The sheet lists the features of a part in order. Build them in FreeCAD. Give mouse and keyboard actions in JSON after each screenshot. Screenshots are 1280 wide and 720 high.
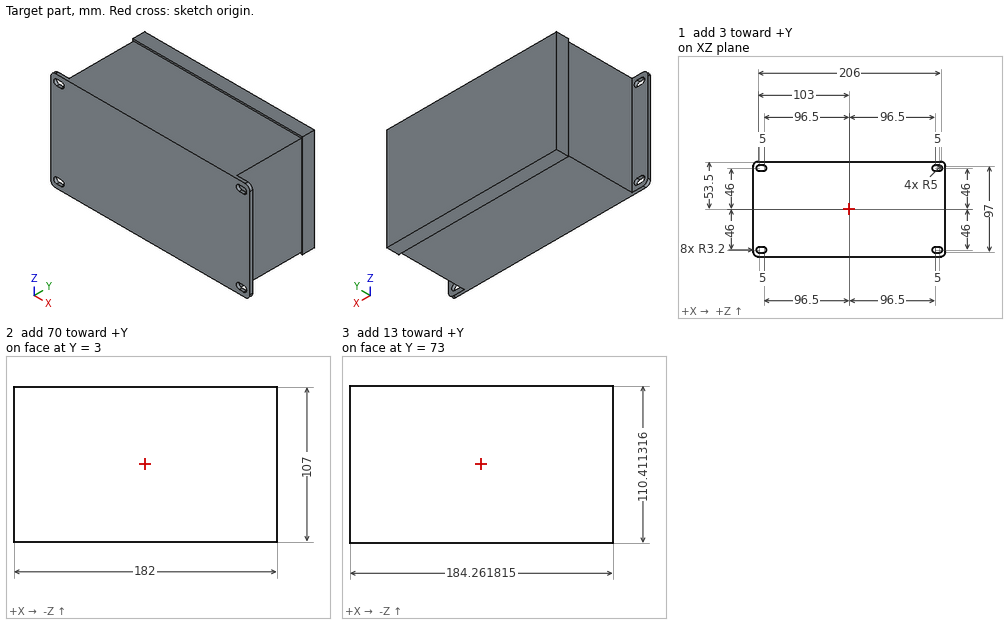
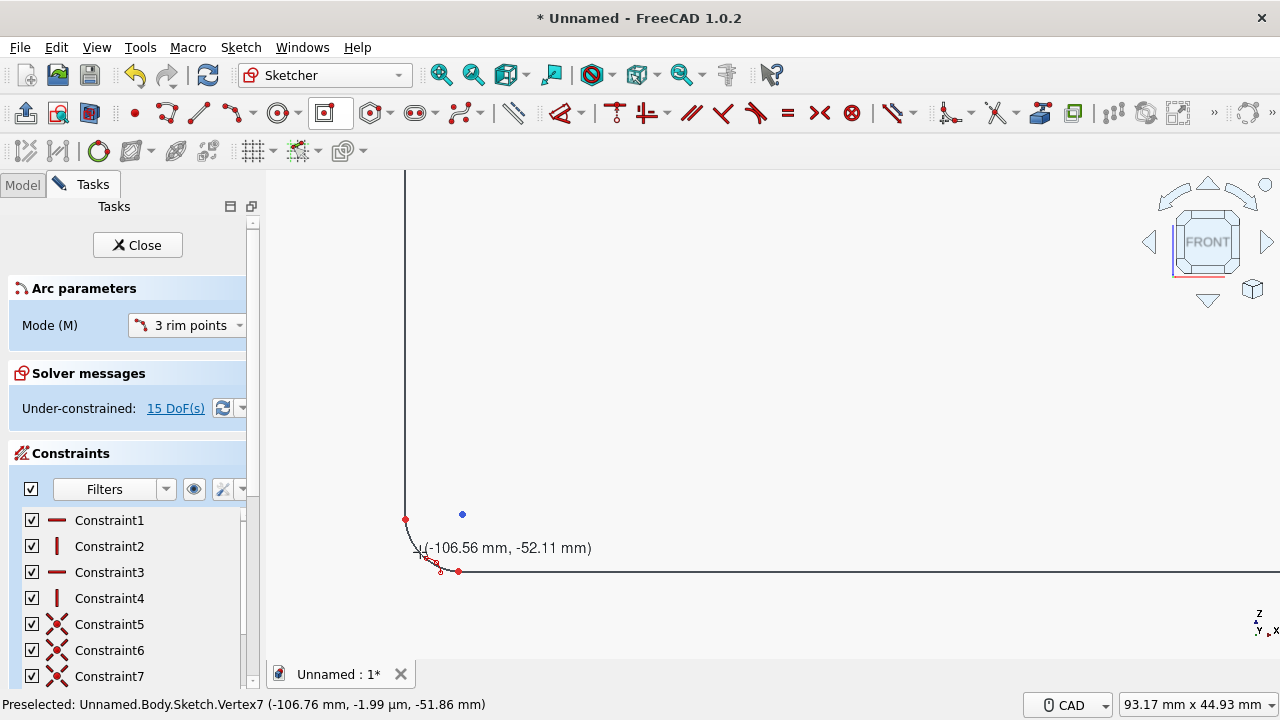
{"action": "scroll", "coordinate": [418, 555], "scroll_direction": "down", "scroll_amount": 7}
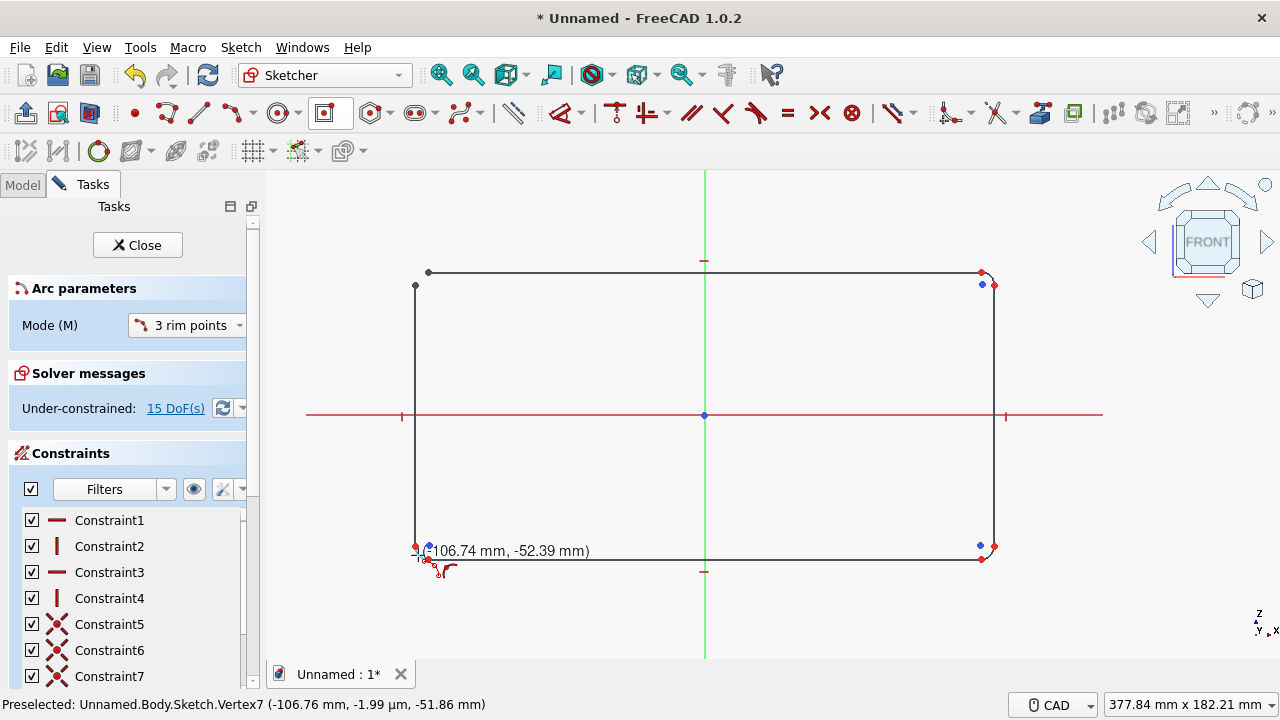
{"action": "left_click", "coordinate": [415, 286]}
{"action": "left_click", "coordinate": [428, 273]}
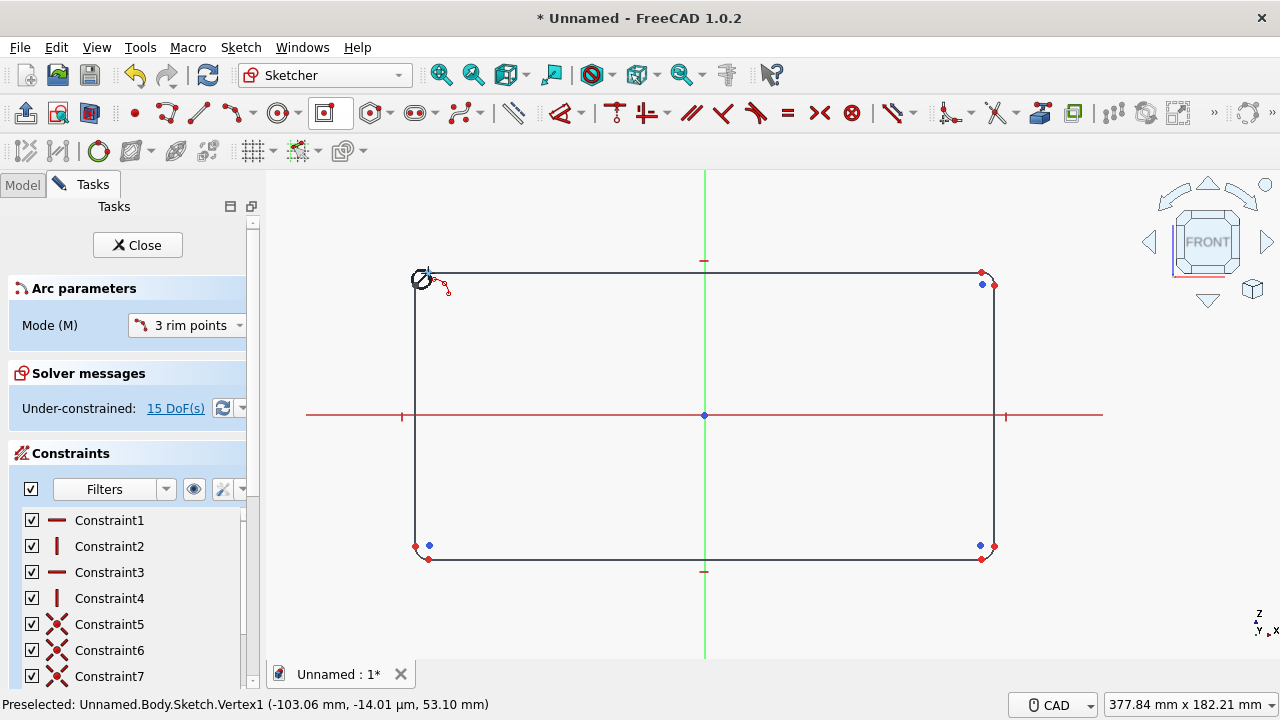
{"action": "scroll", "coordinate": [419, 276], "scroll_direction": "up", "scroll_amount": 7}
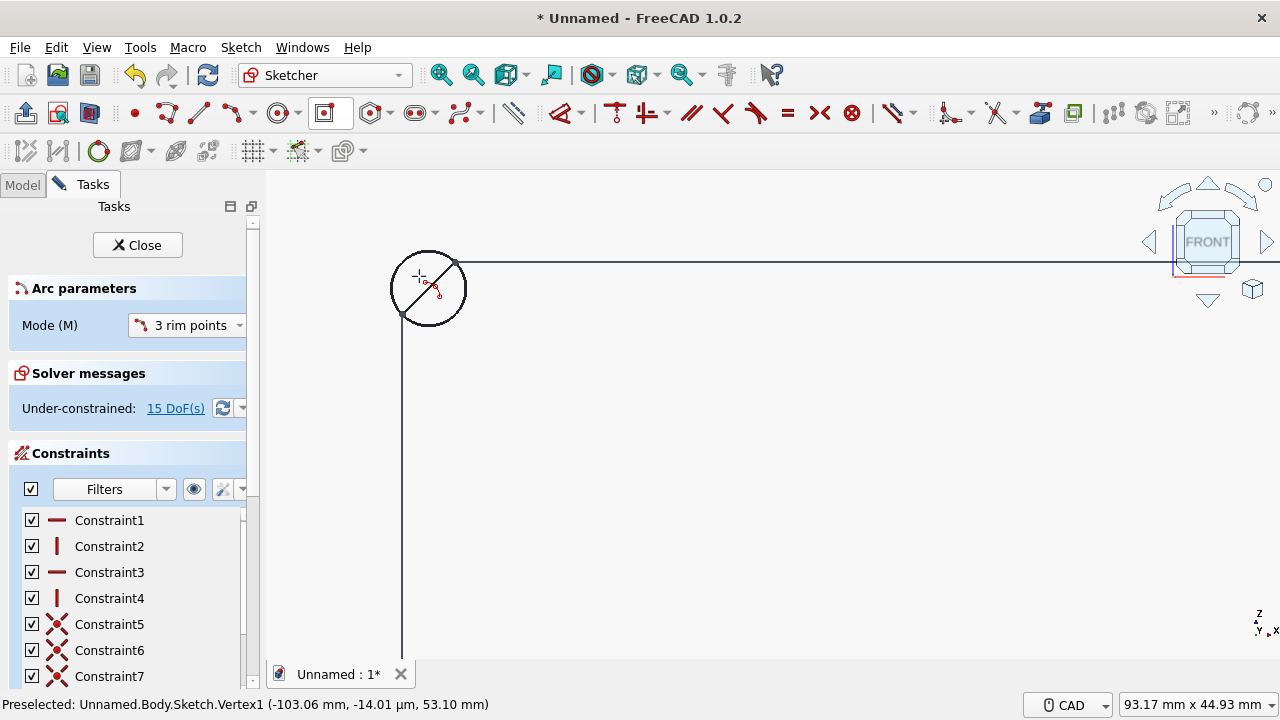
{"action": "left_click", "coordinate": [417, 274]}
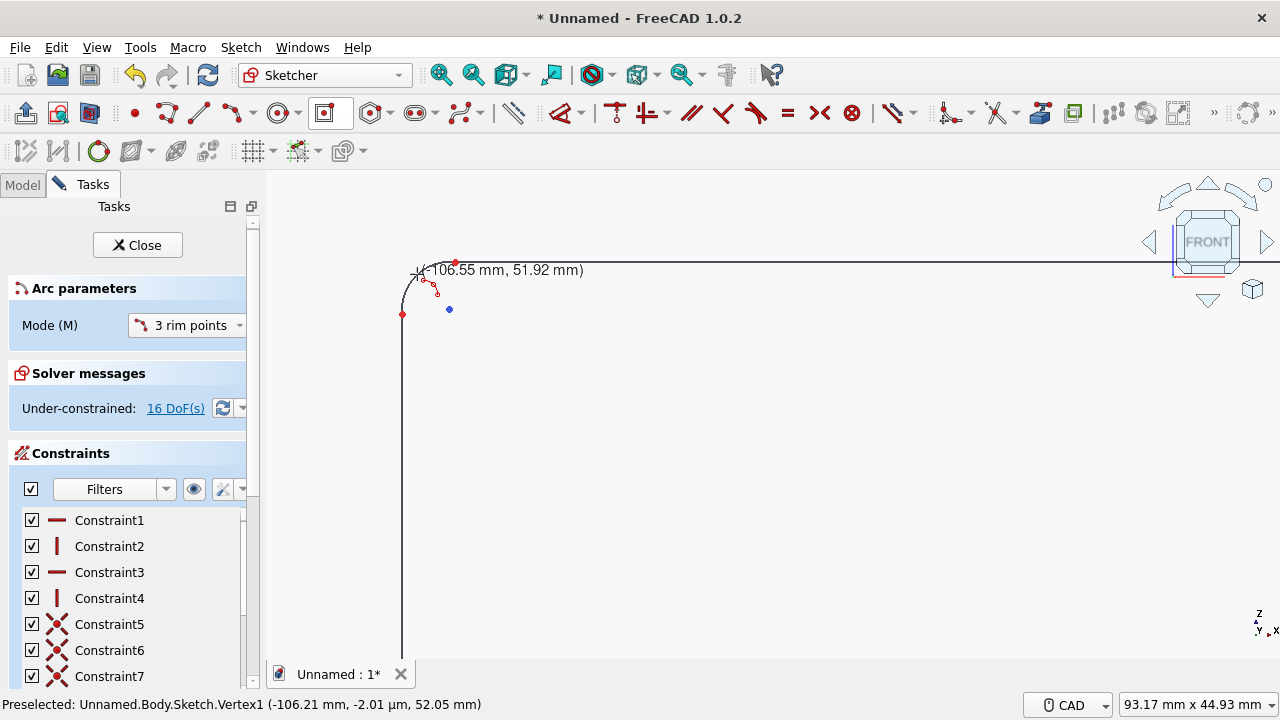
{"action": "left_click", "coordinate": [416, 114]}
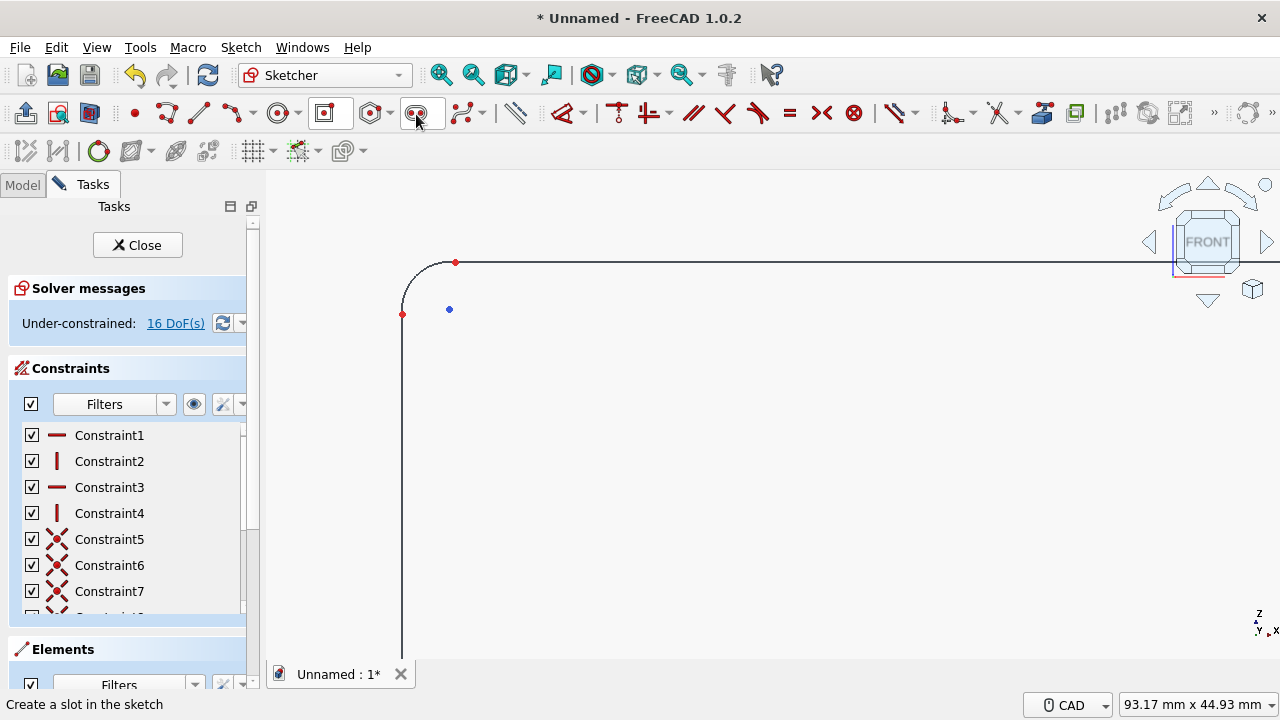
{"action": "left_click", "coordinate": [472, 339]}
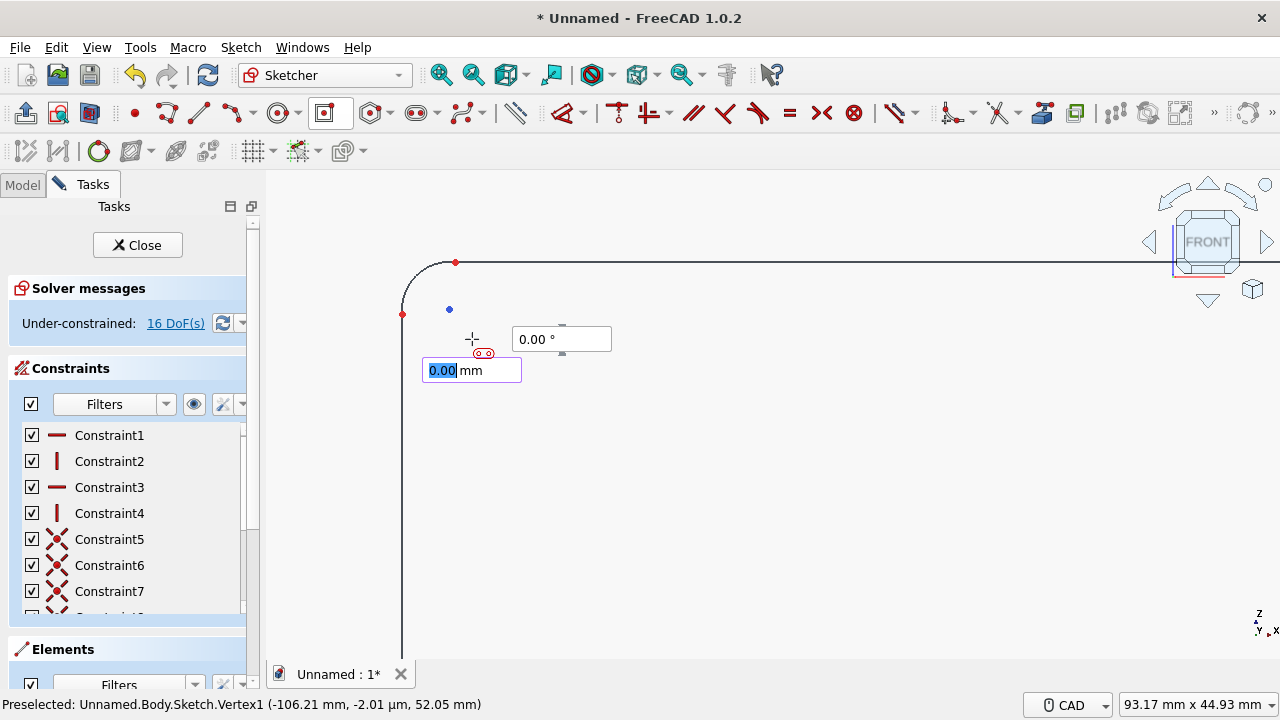
{"action": "scroll", "coordinate": [419, 275], "scroll_direction": "down", "scroll_amount": 7}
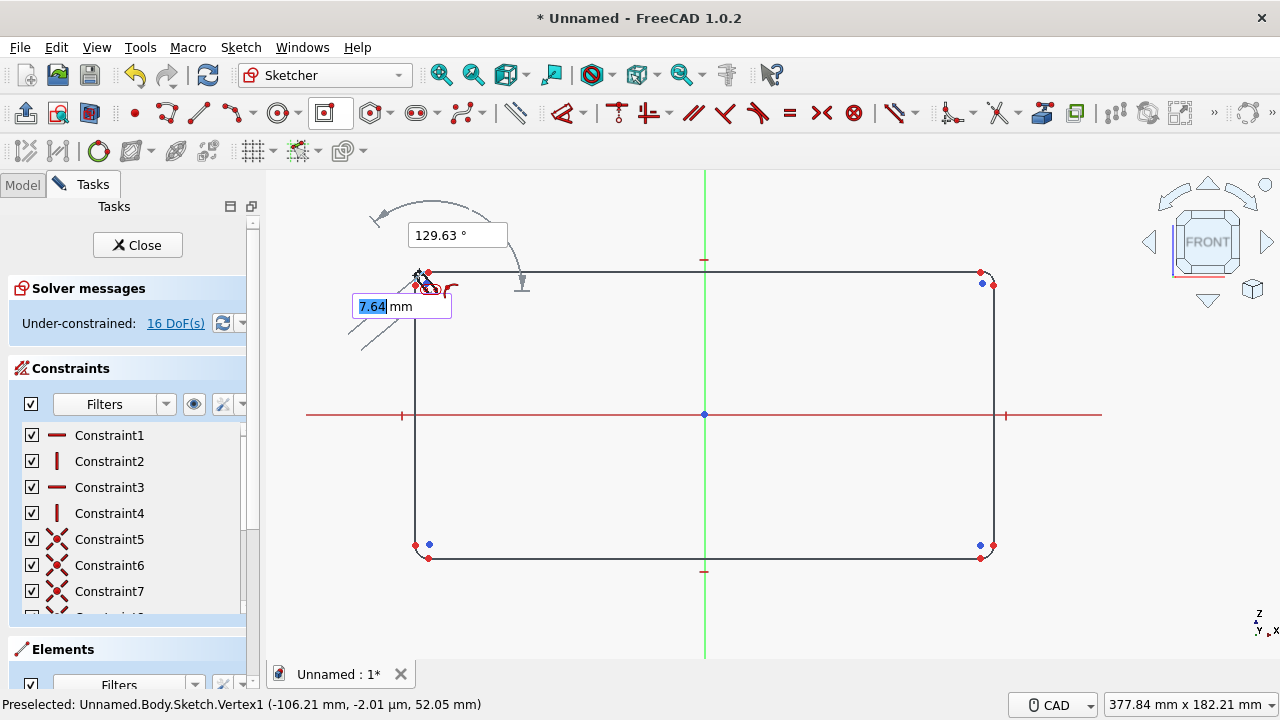
{"action": "left_click", "coordinate": [446, 291]}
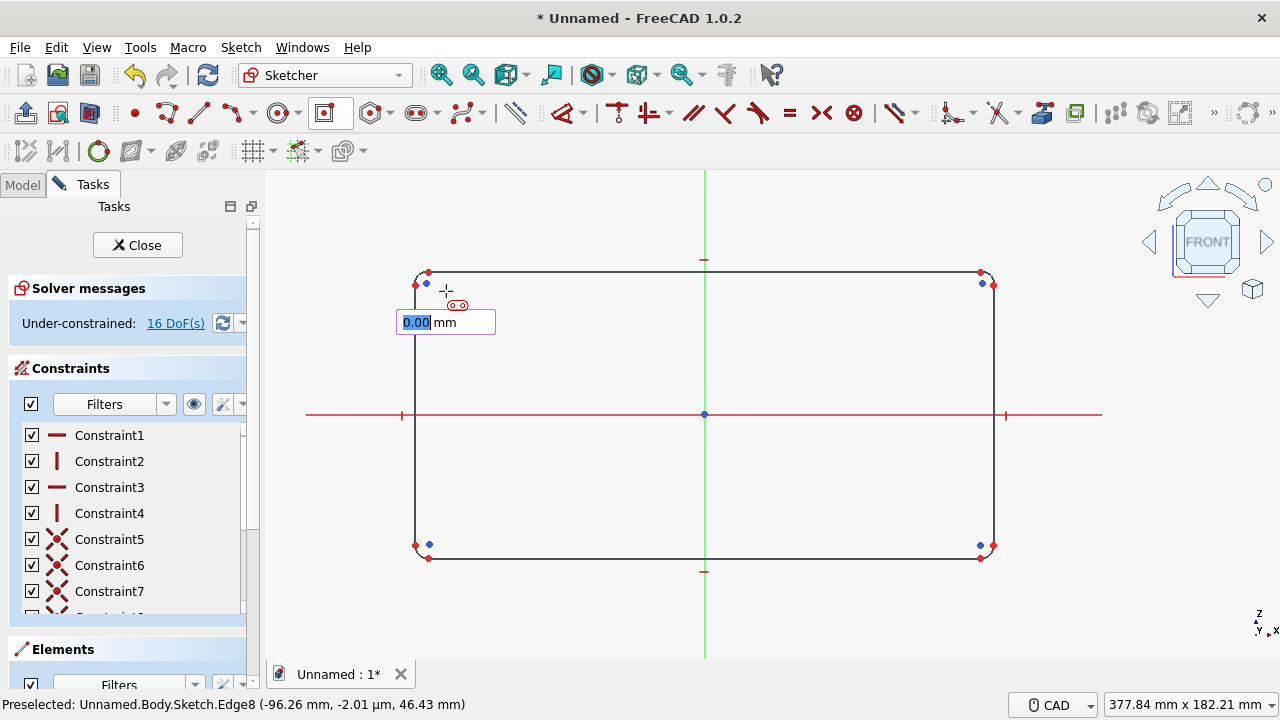
{"action": "scroll", "coordinate": [439, 300], "scroll_direction": "up", "scroll_amount": 4}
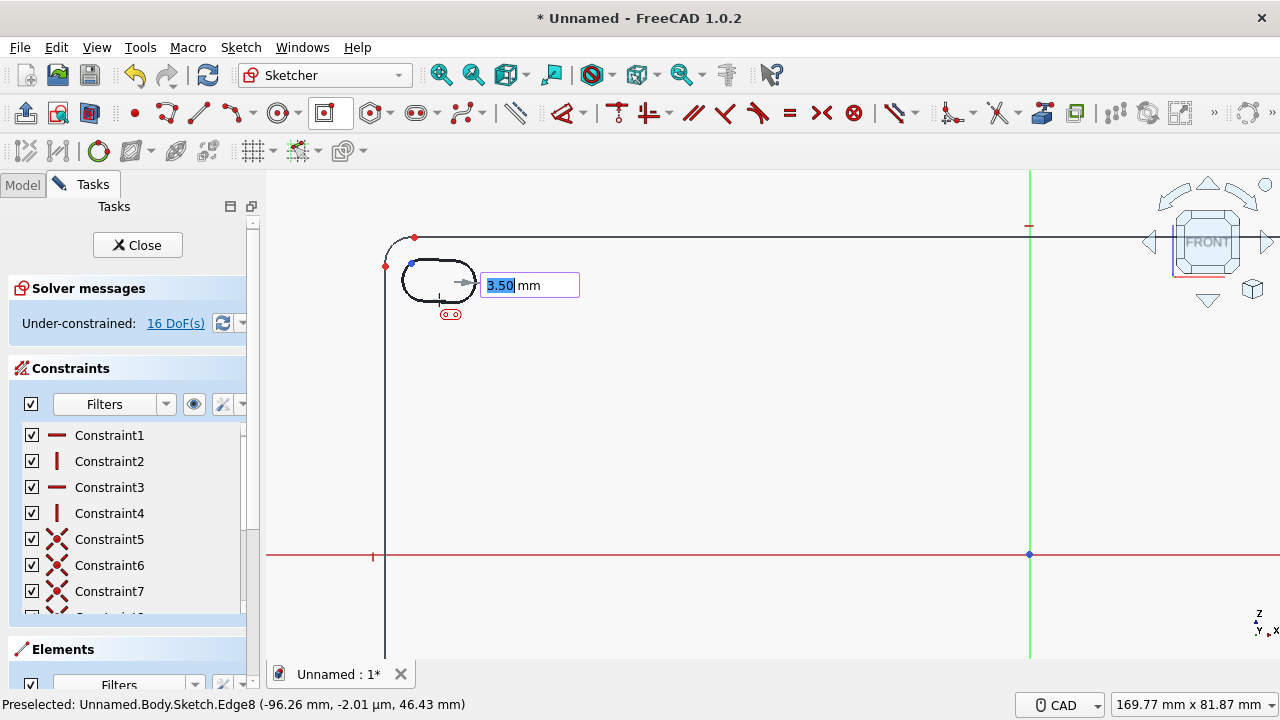
{"action": "left_click", "coordinate": [439, 299]}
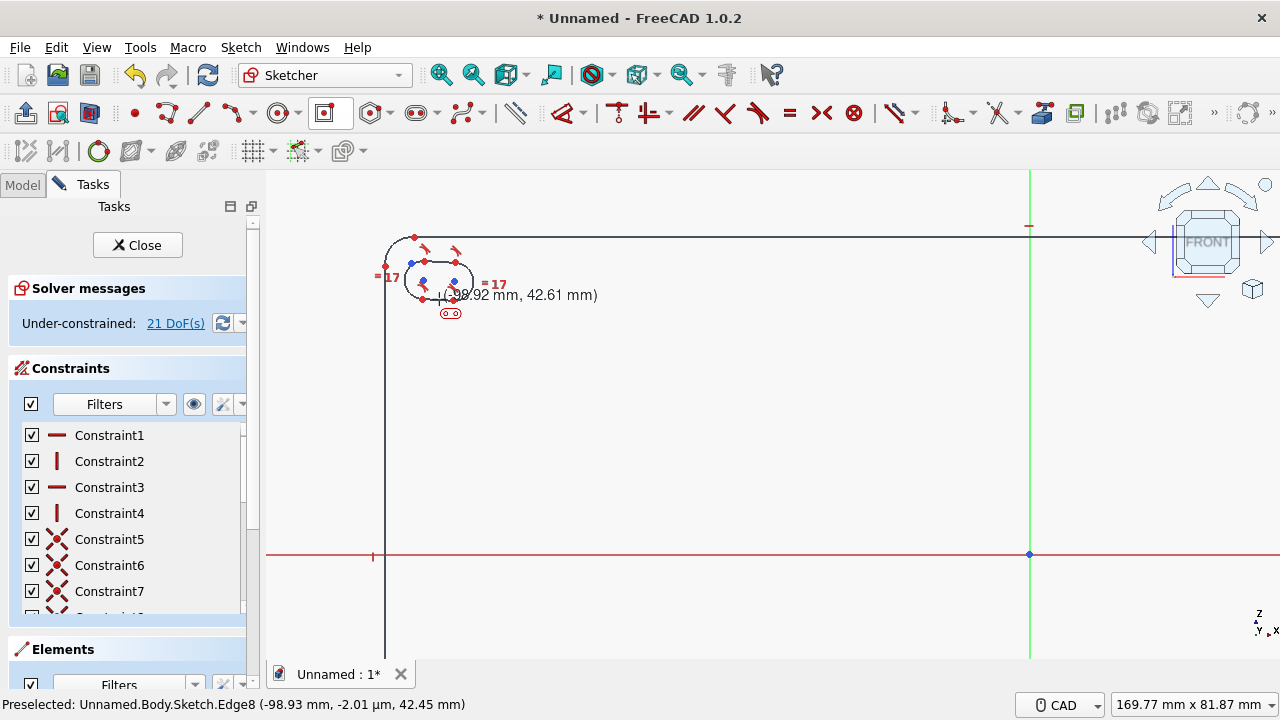
{"action": "scroll", "coordinate": [439, 300], "scroll_direction": "down", "scroll_amount": 4}